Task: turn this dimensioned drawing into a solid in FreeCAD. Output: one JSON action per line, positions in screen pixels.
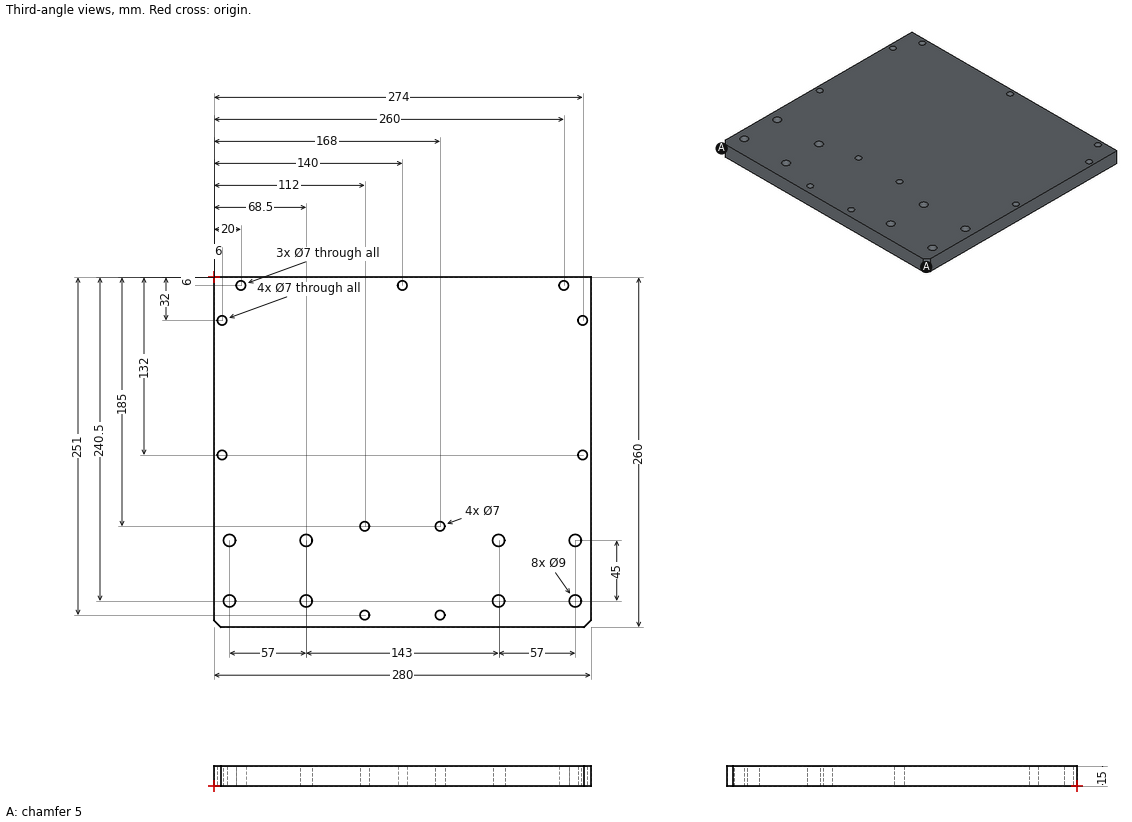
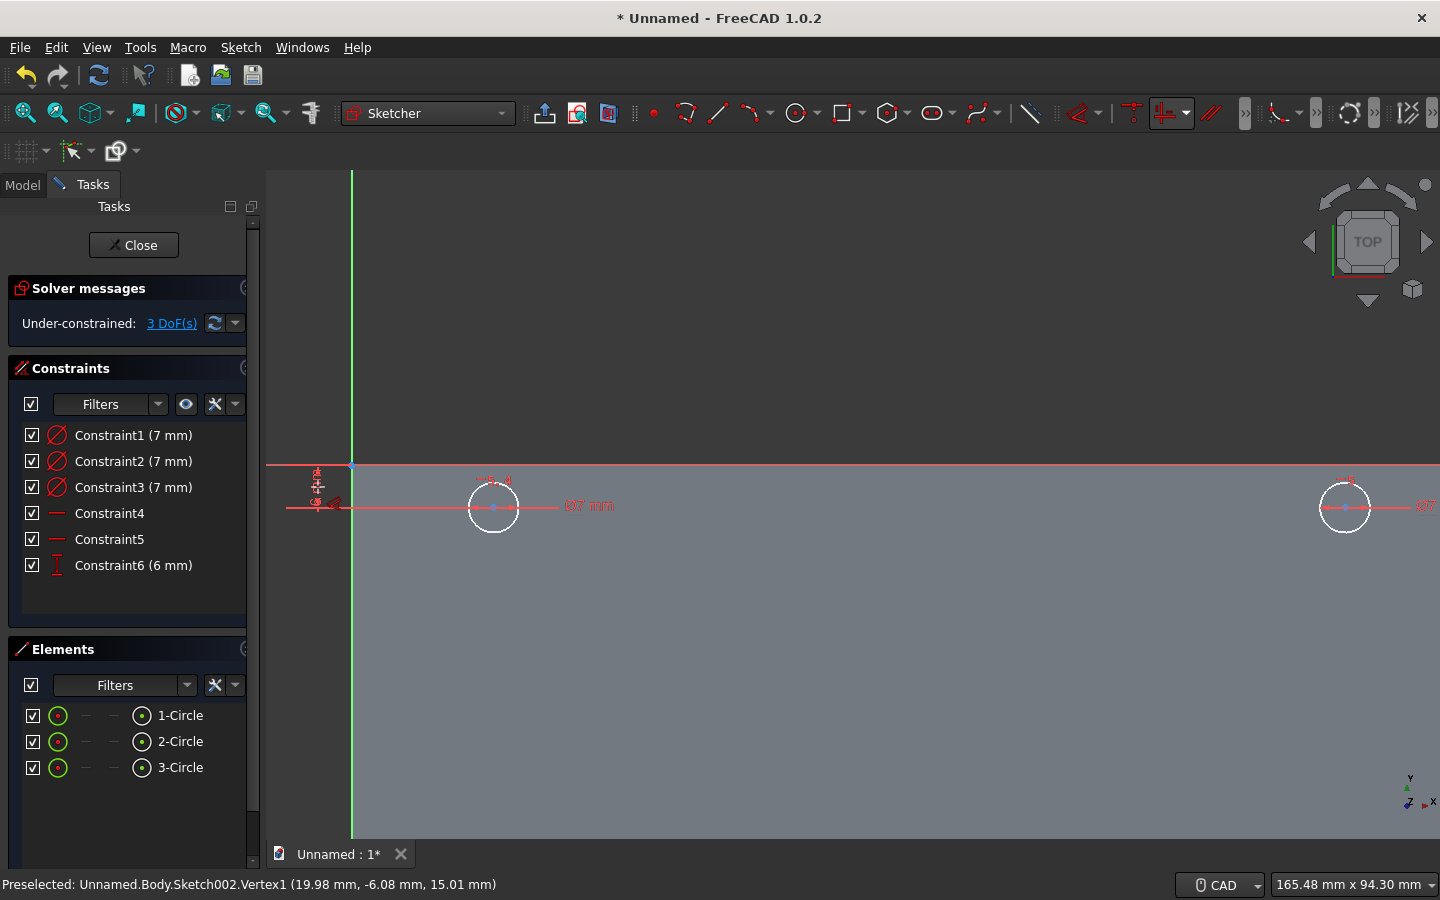
{"action": "left_click", "coordinate": [494, 508]}
{"action": "left_click", "coordinate": [423, 431]}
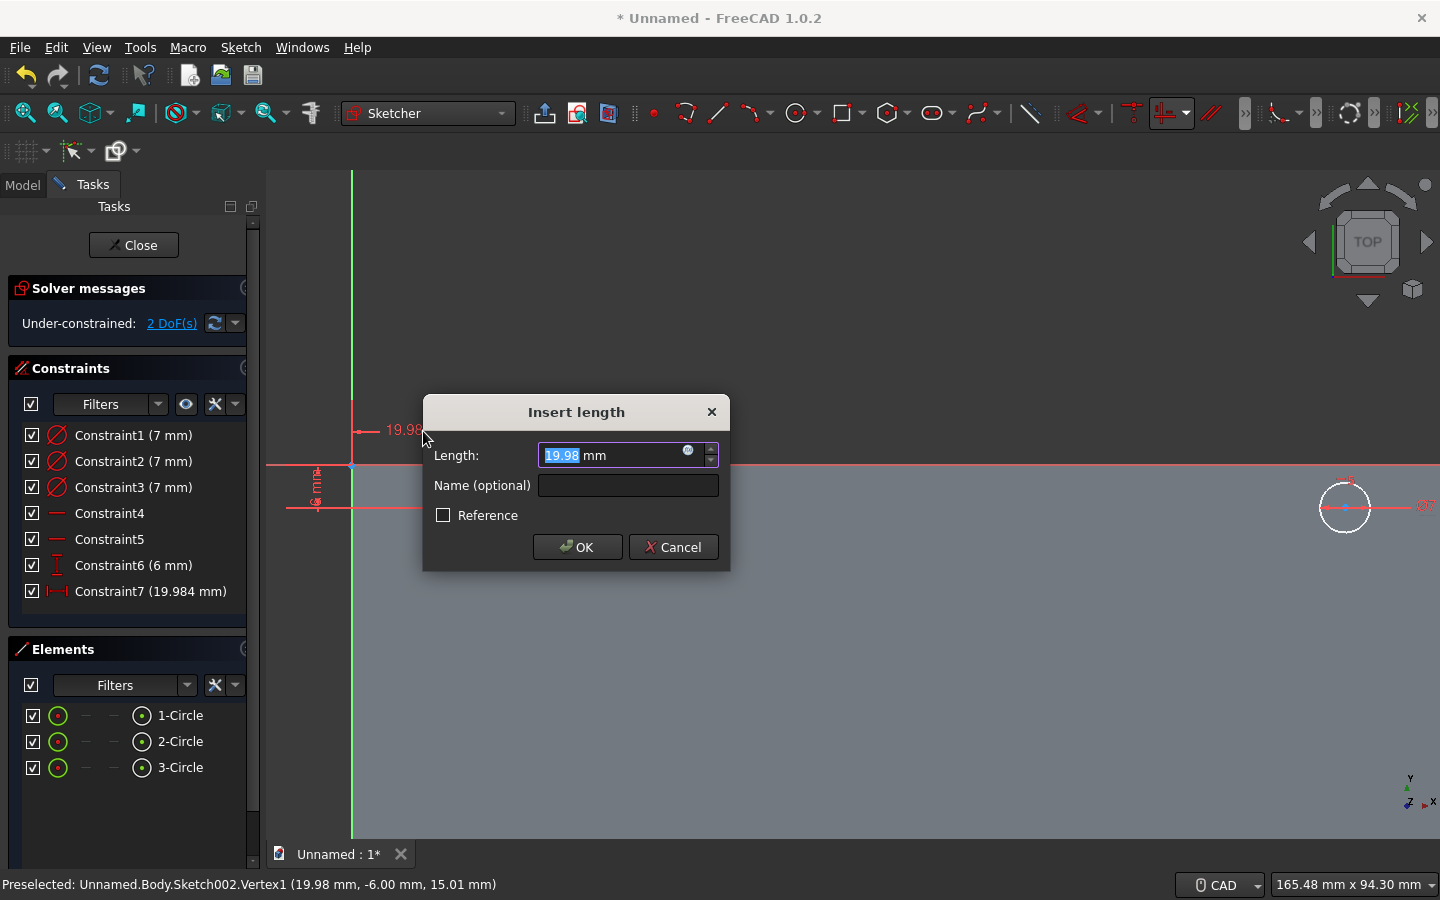
{"action": "type", "text": "20"}
{"action": "key", "text": "Return"}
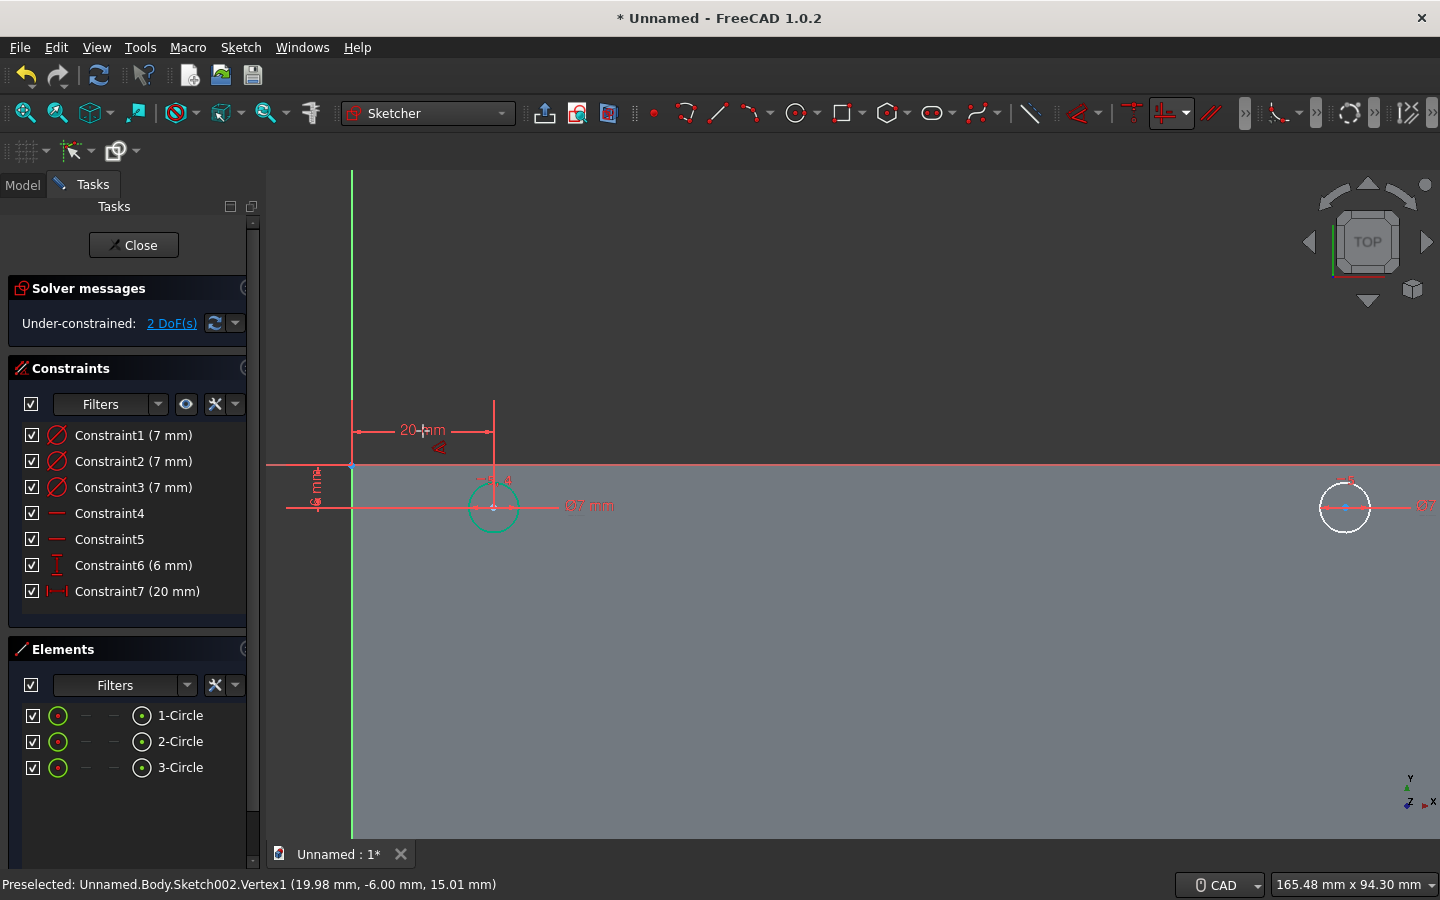
{"action": "scroll", "coordinate": [492, 508], "scroll_direction": "down", "scroll_amount": 5}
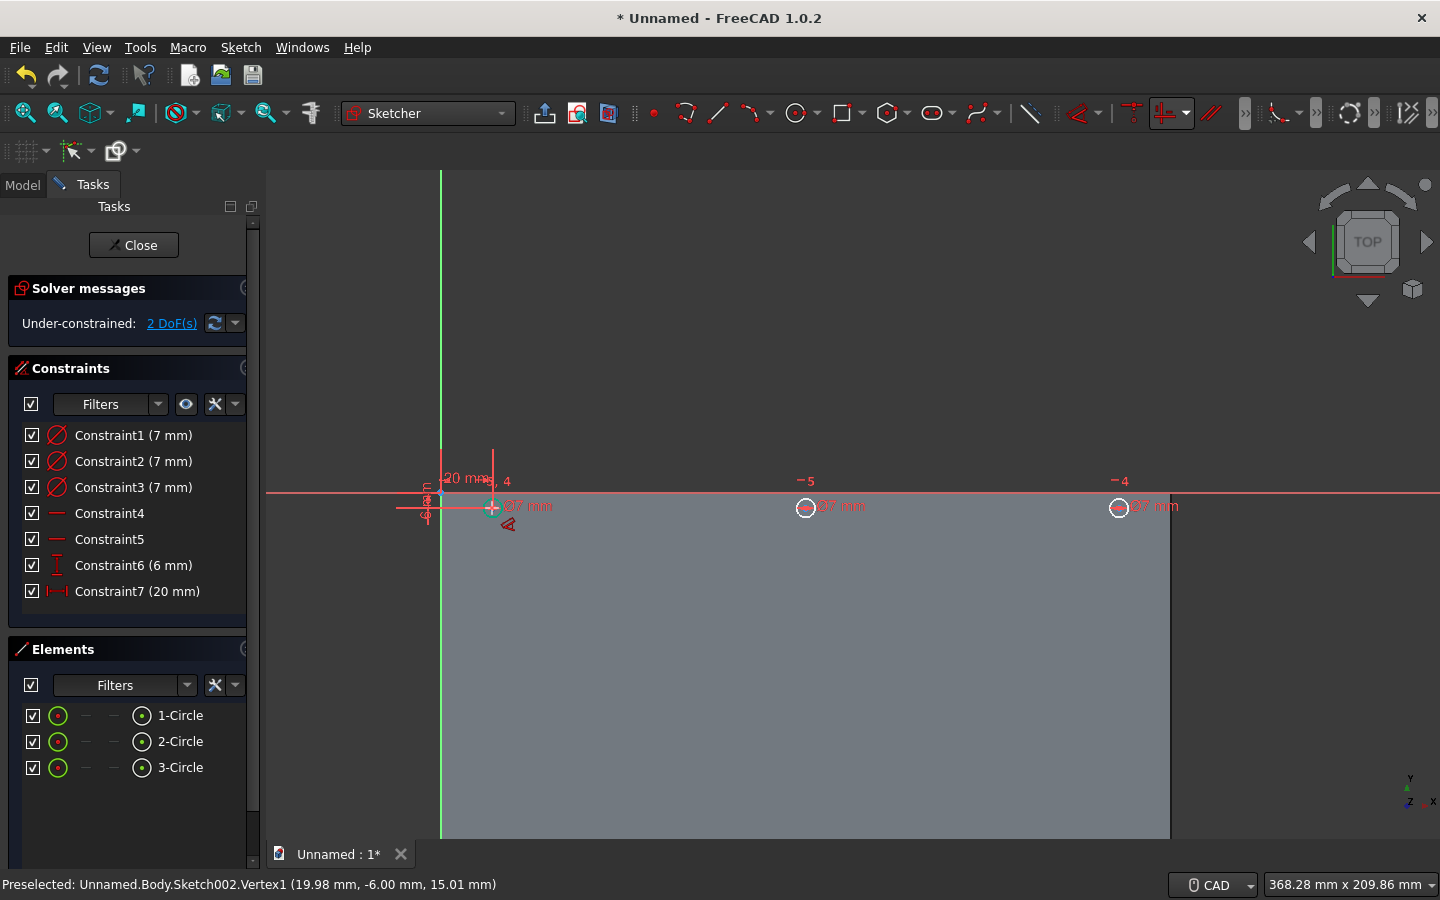
{"action": "left_click", "coordinate": [1119, 508]}
{"action": "left_click", "coordinate": [780, 459]}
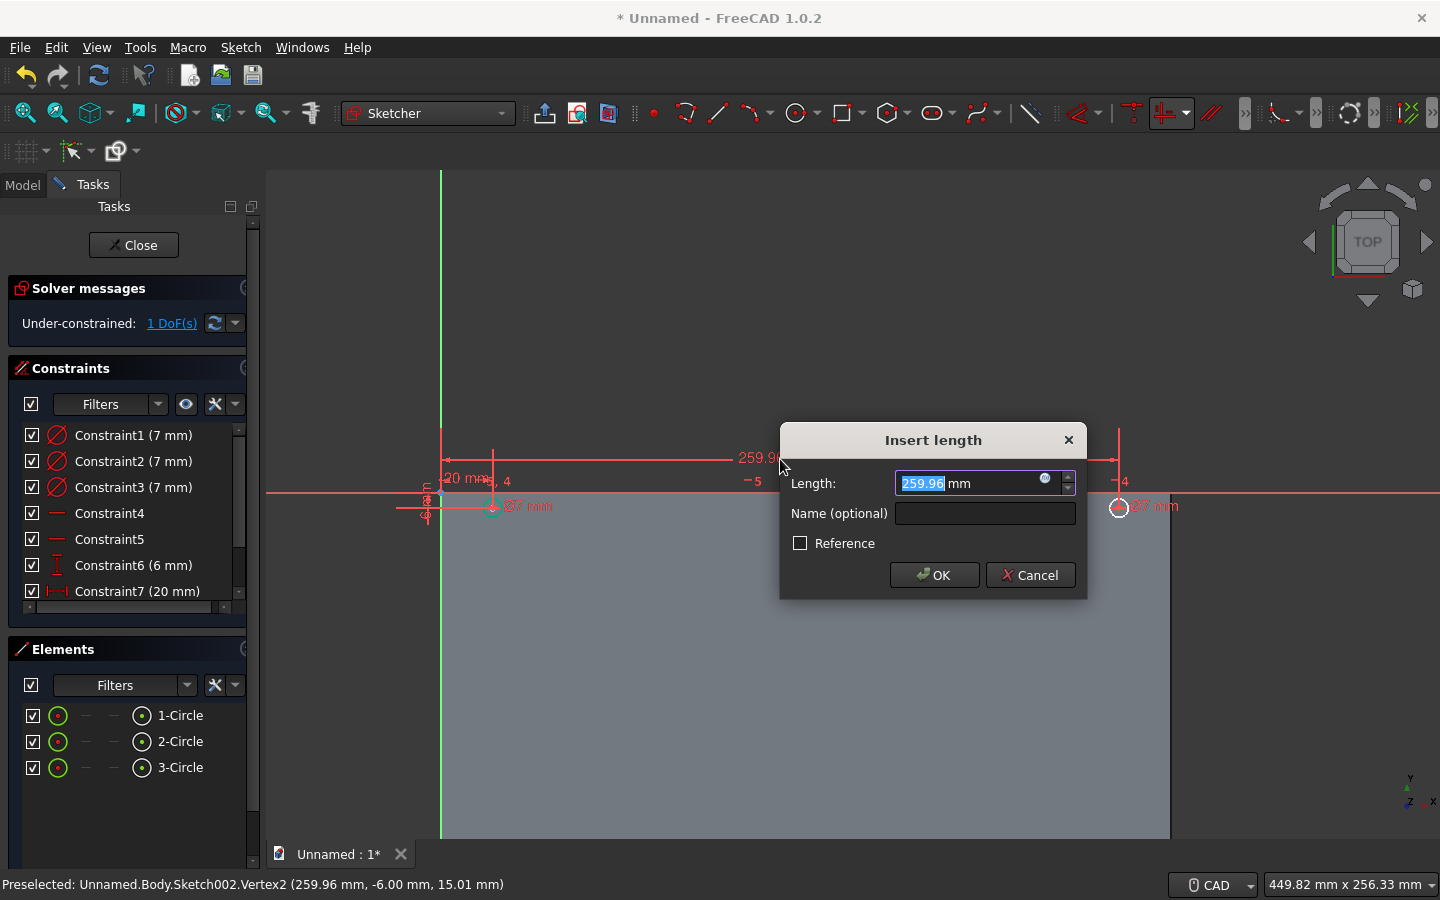
{"action": "type", "text": "260"}
{"action": "key", "text": "Return"}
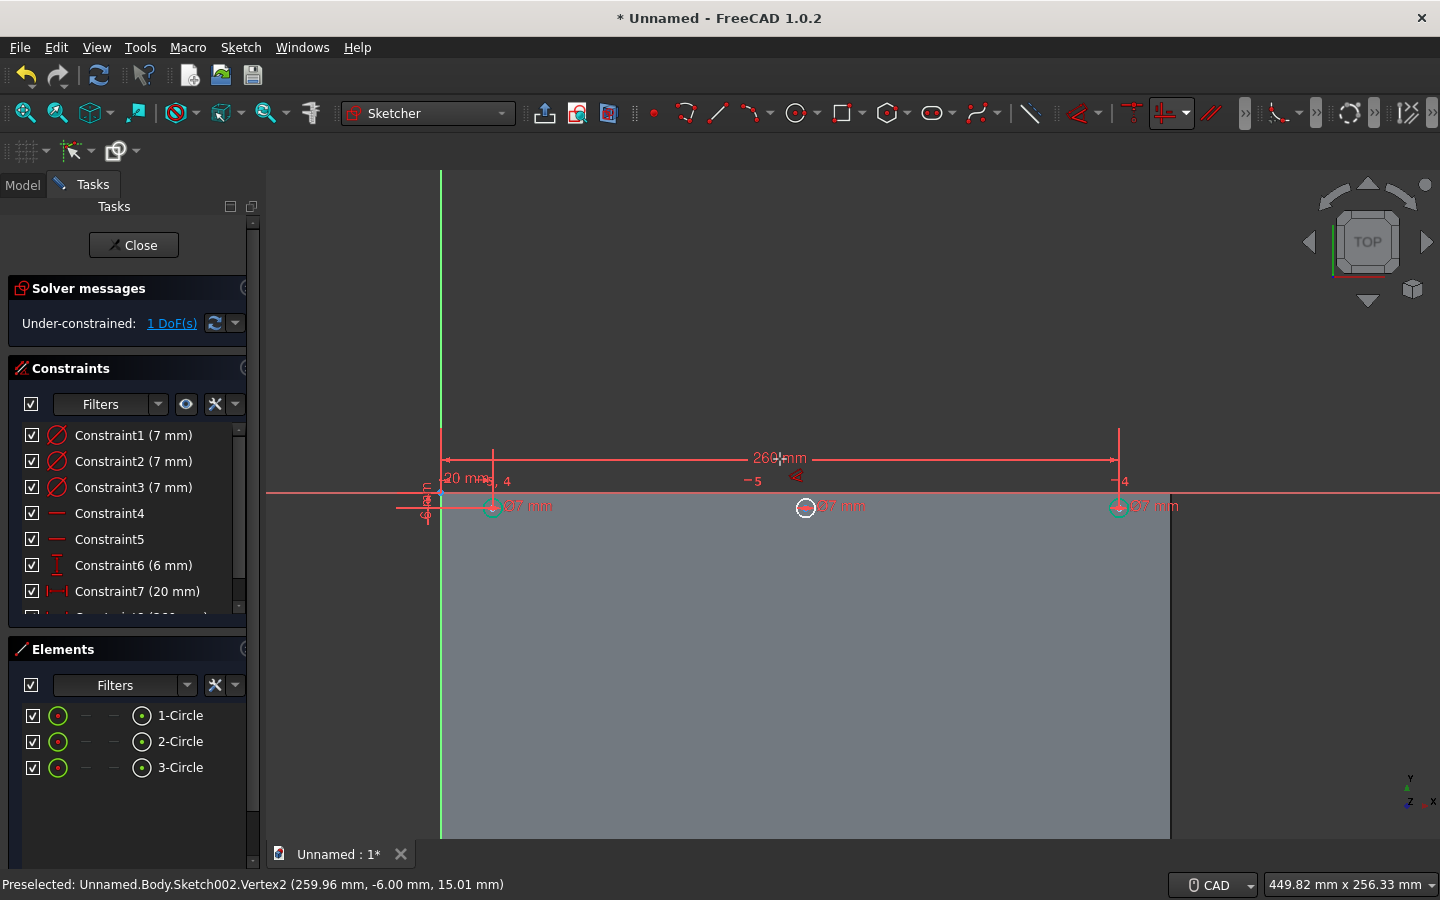
{"action": "left_click", "coordinate": [806, 508]}
{"action": "left_click", "coordinate": [623, 459]}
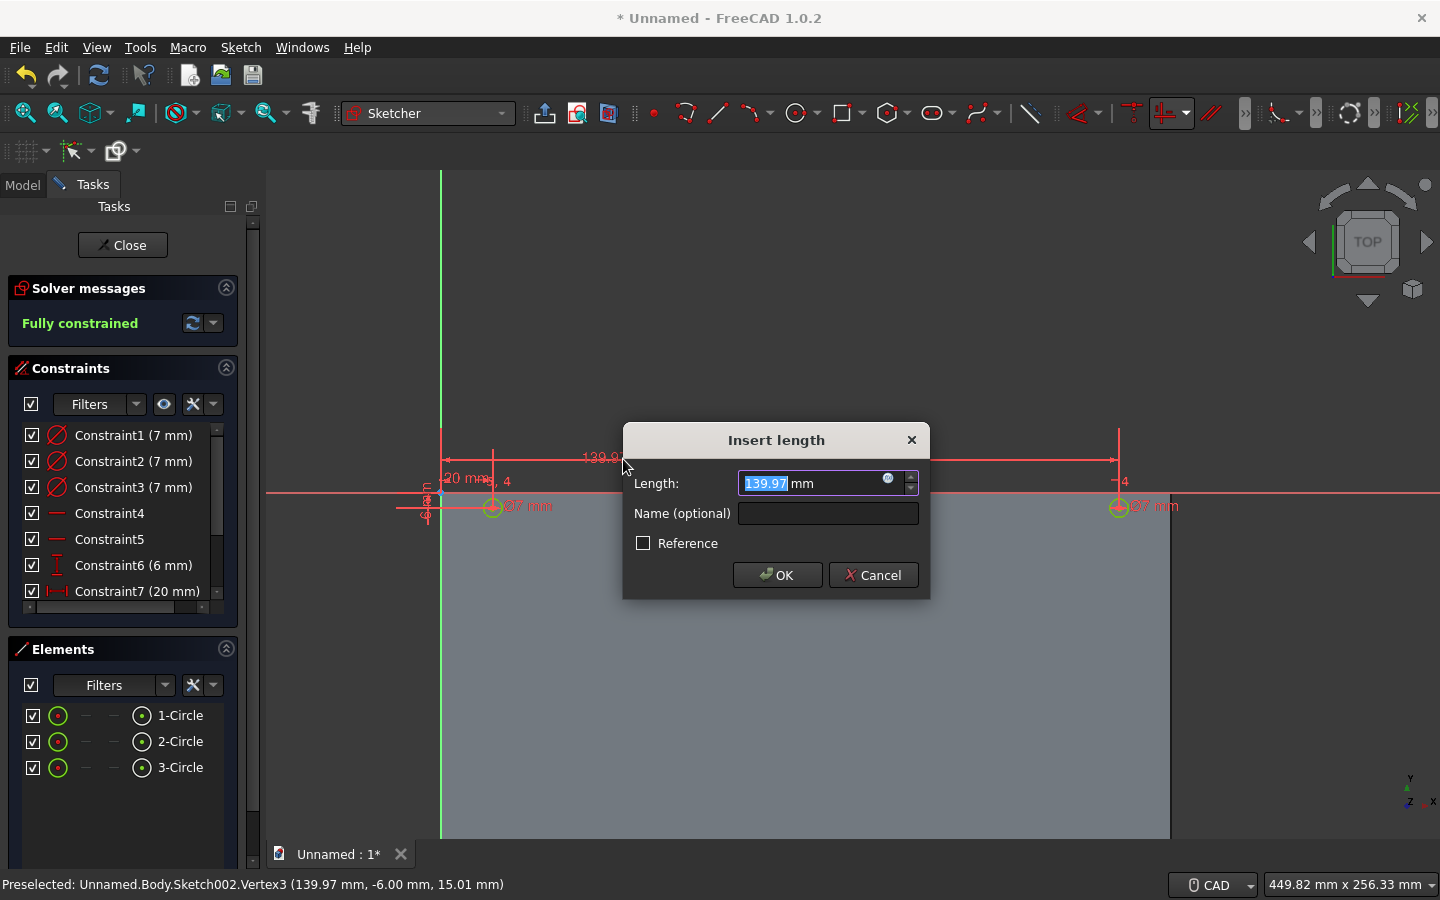
{"action": "type", "text": "140"}
{"action": "key", "text": "Return"}
{"action": "key", "text": "Escape"}